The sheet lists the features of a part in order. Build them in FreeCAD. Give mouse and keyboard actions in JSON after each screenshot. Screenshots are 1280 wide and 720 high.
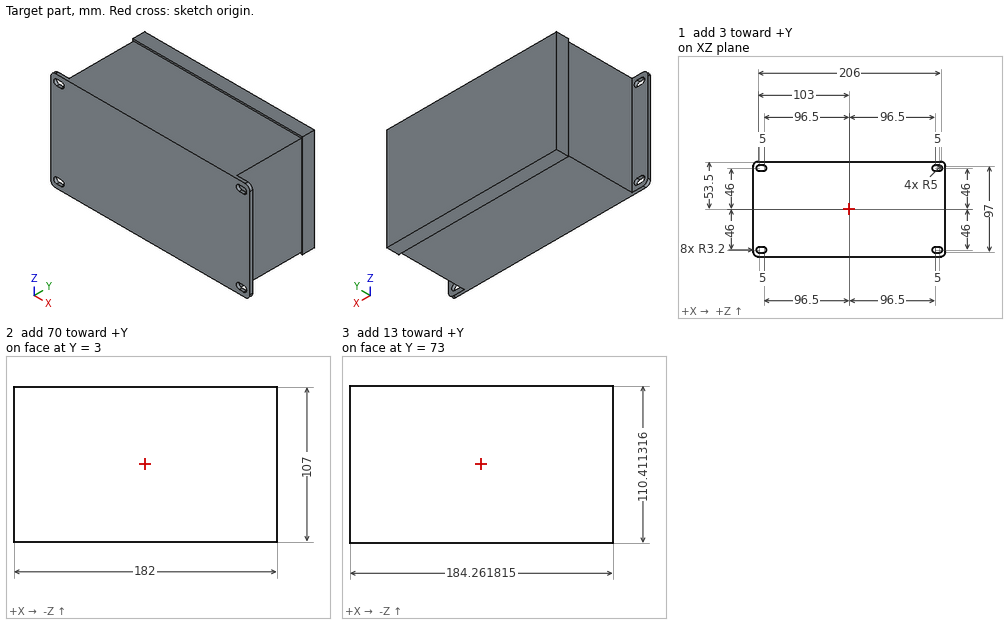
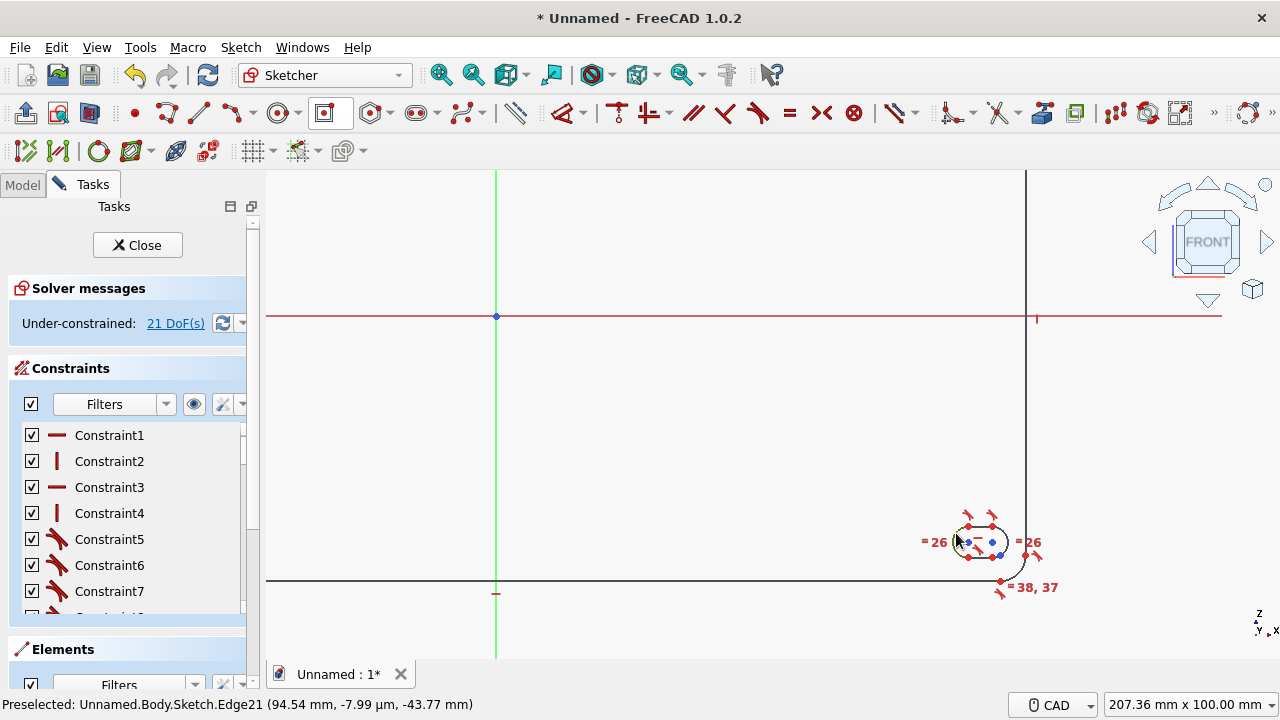
{"action": "key", "text": "e"}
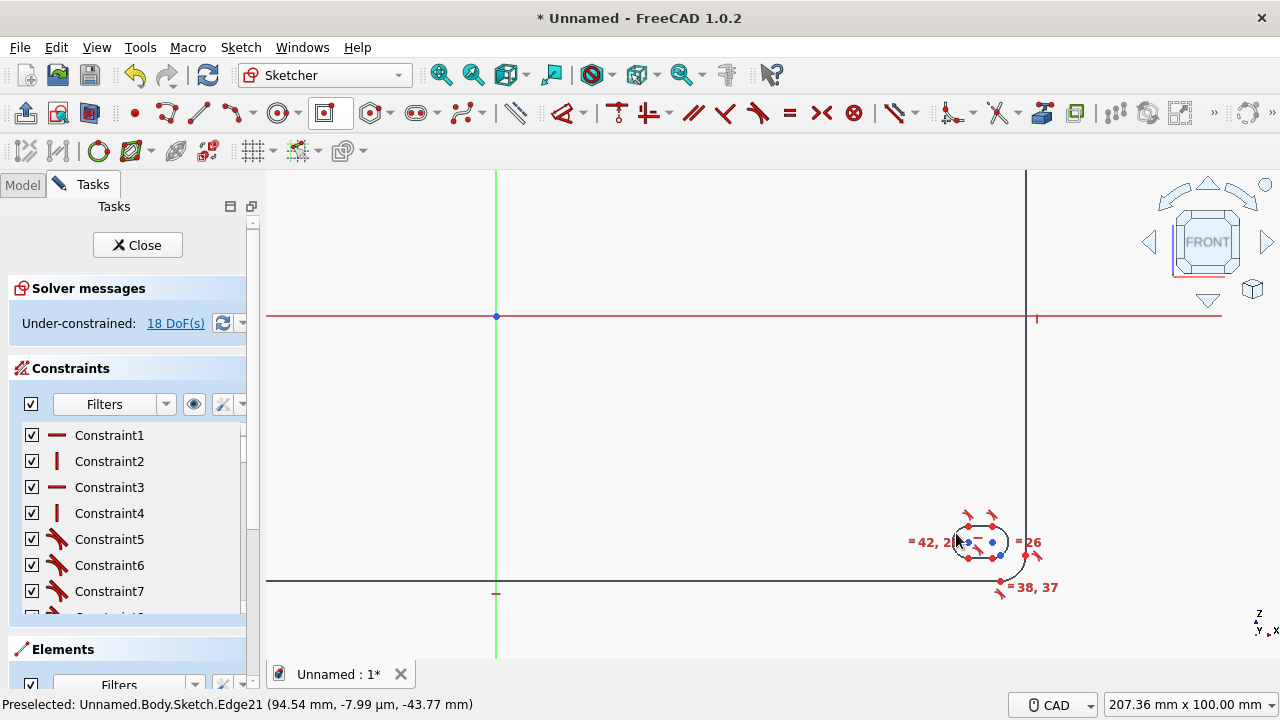
{"action": "left_click", "coordinate": [562, 114]}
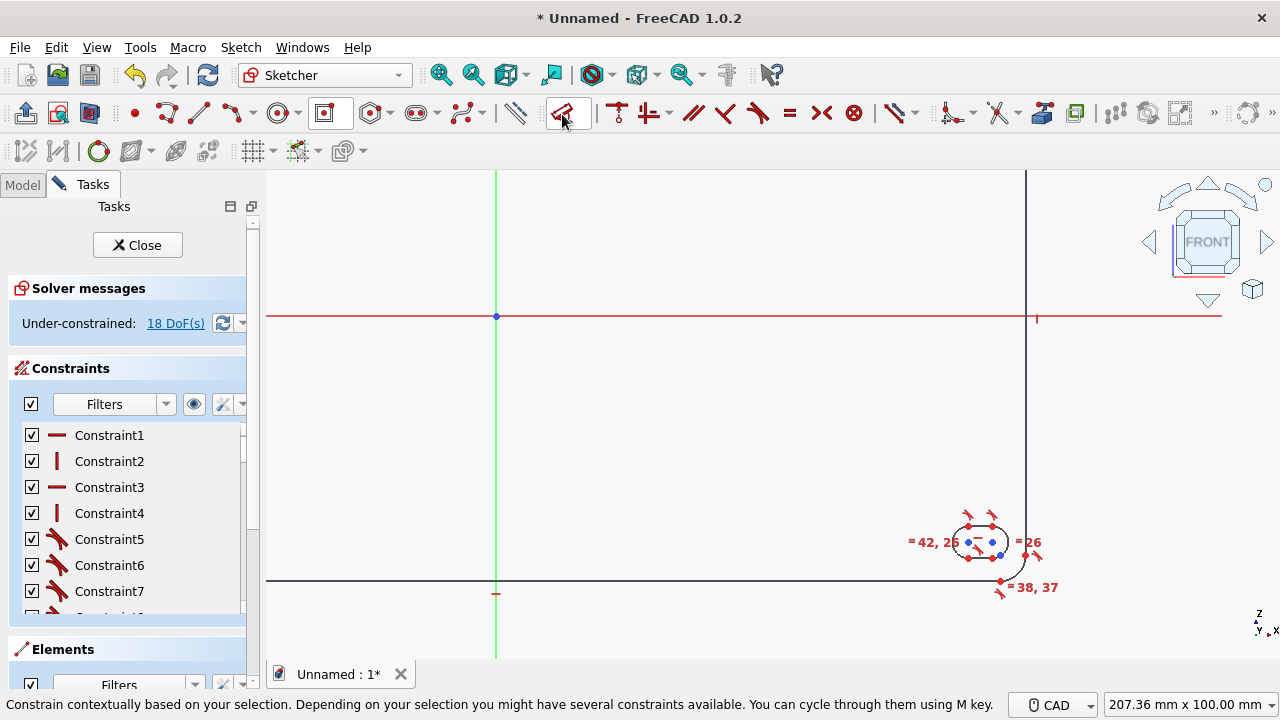
{"action": "scroll", "coordinate": [958, 534], "scroll_direction": "down", "scroll_amount": 3}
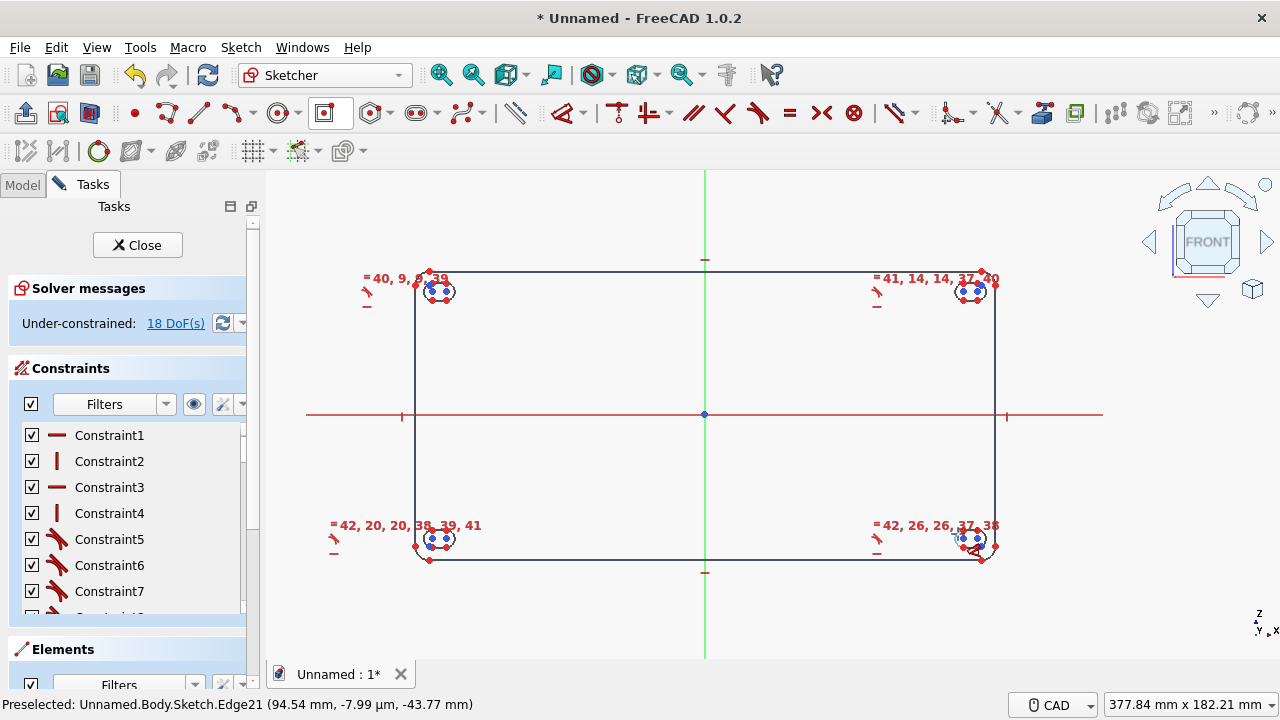
{"action": "scroll", "coordinate": [994, 279], "scroll_direction": "up", "scroll_amount": 6}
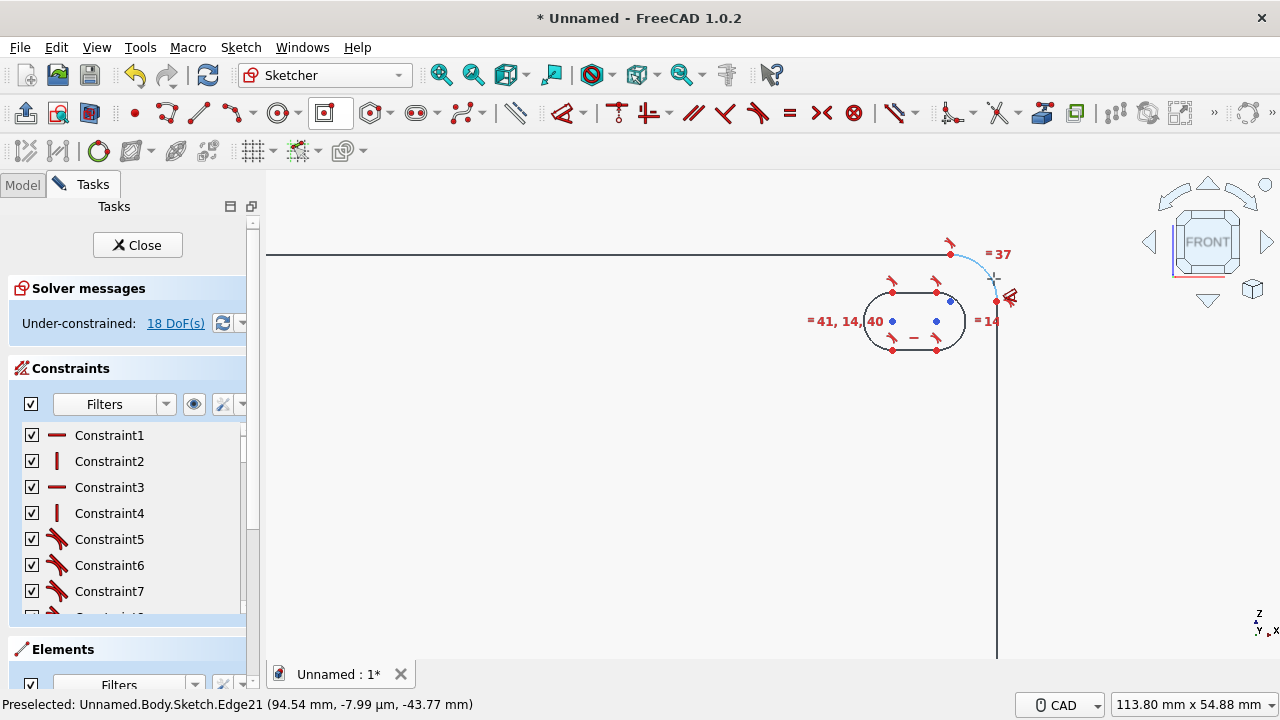
{"action": "left_click", "coordinate": [992, 280]}
{"action": "left_click", "coordinate": [1021, 265]}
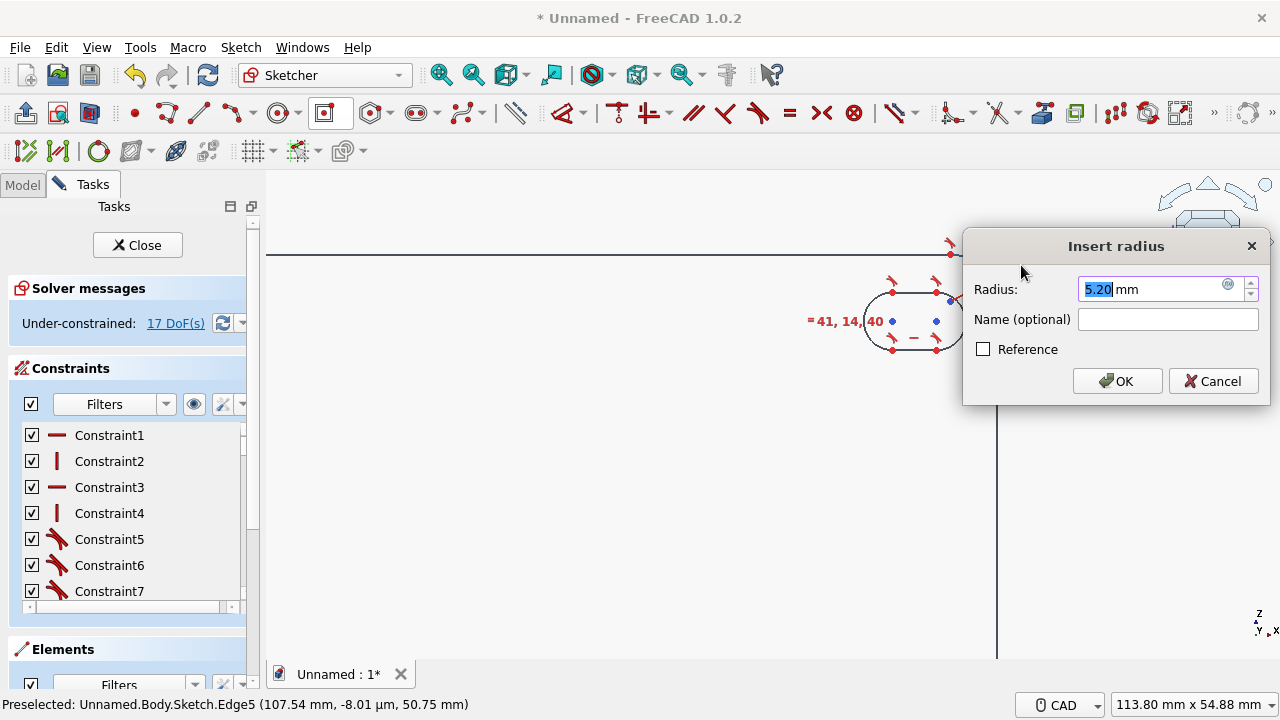
{"action": "type", "text": "5"}
{"action": "key", "text": "Return"}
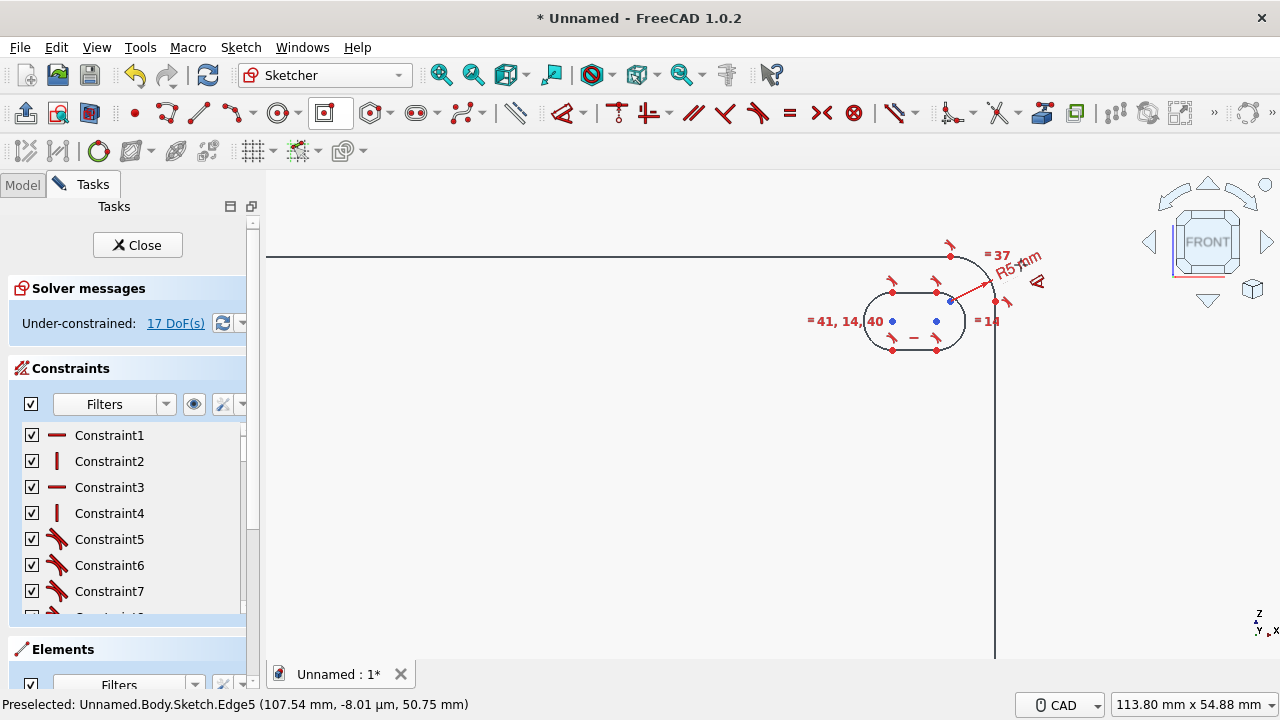
{"action": "scroll", "coordinate": [994, 279], "scroll_direction": "down", "scroll_amount": 6}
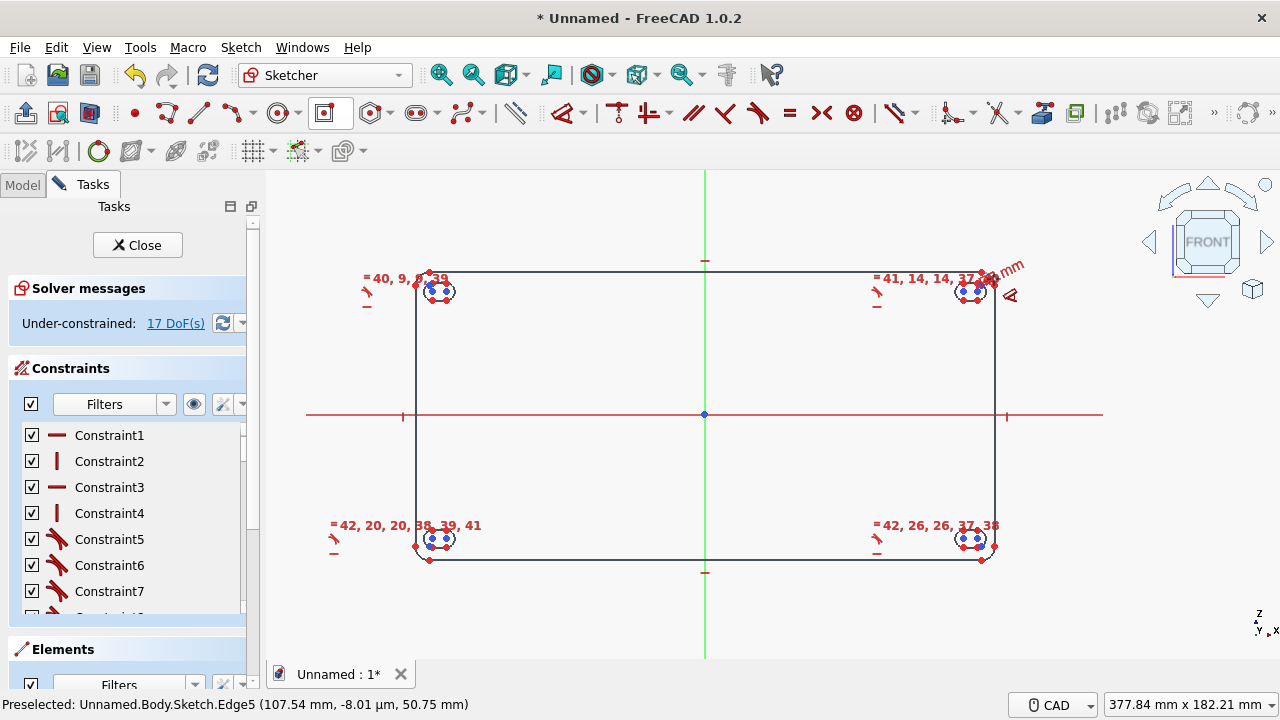
{"action": "scroll", "coordinate": [426, 287], "scroll_direction": "up", "scroll_amount": 8}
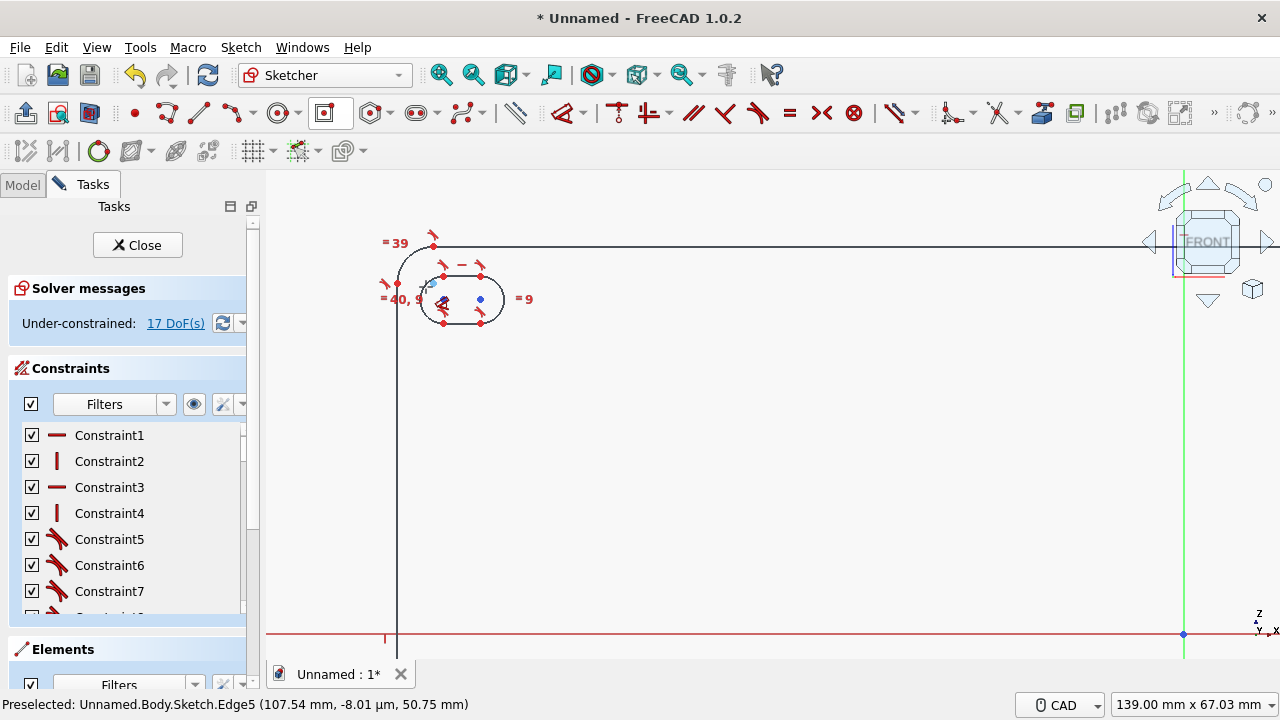
{"action": "left_click", "coordinate": [424, 285]}
{"action": "left_click", "coordinate": [398, 266]}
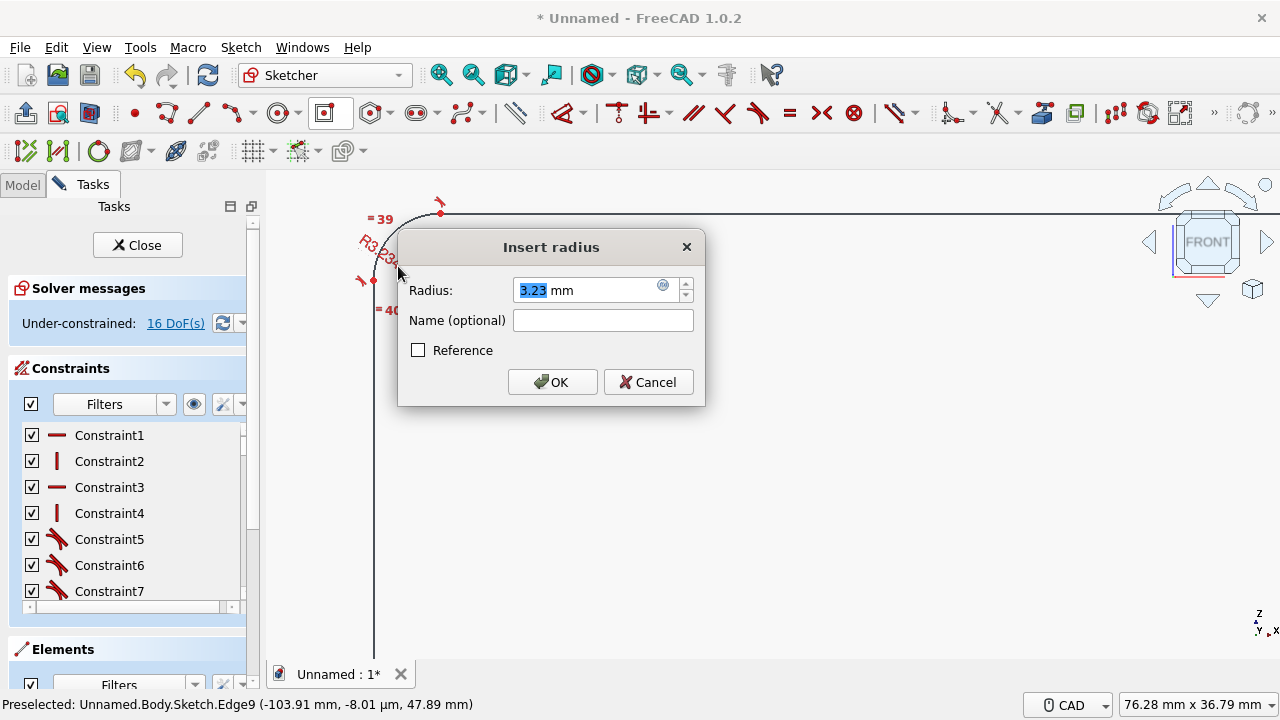
{"action": "type", "text": "3.2"}
{"action": "key", "text": "Return"}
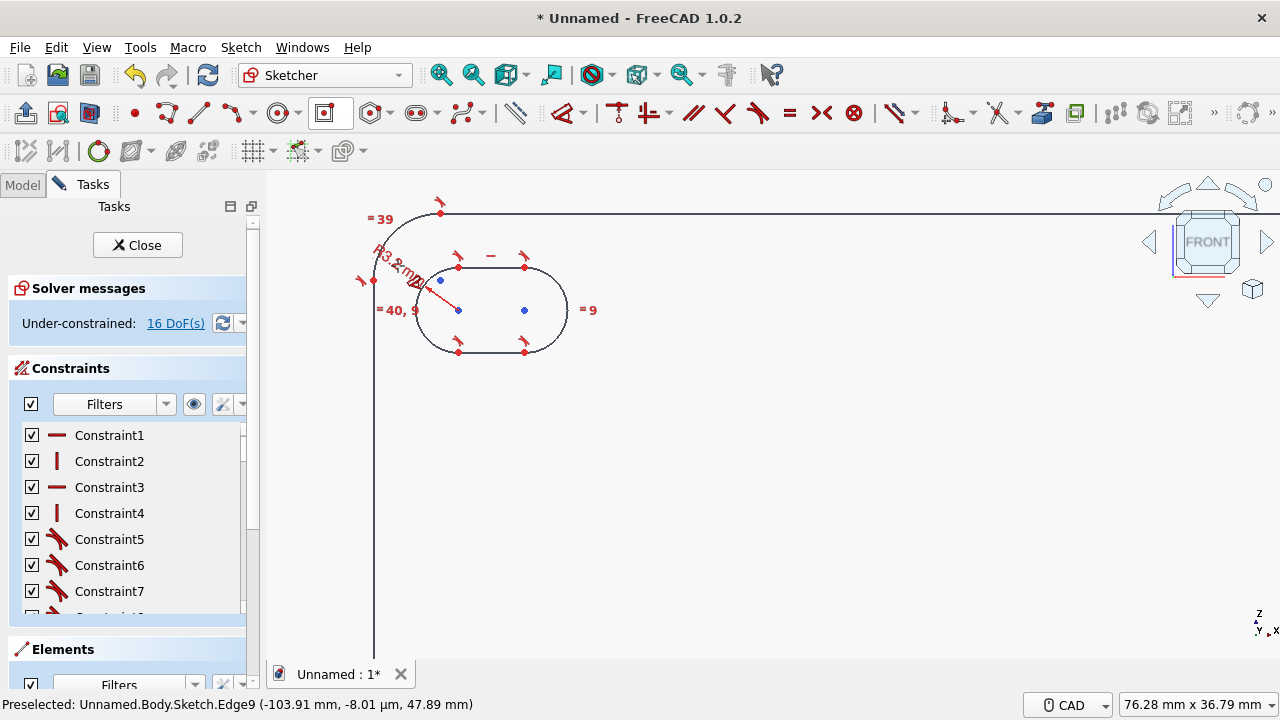
{"action": "left_click", "coordinate": [478, 268]}
{"action": "left_click", "coordinate": [492, 234]}